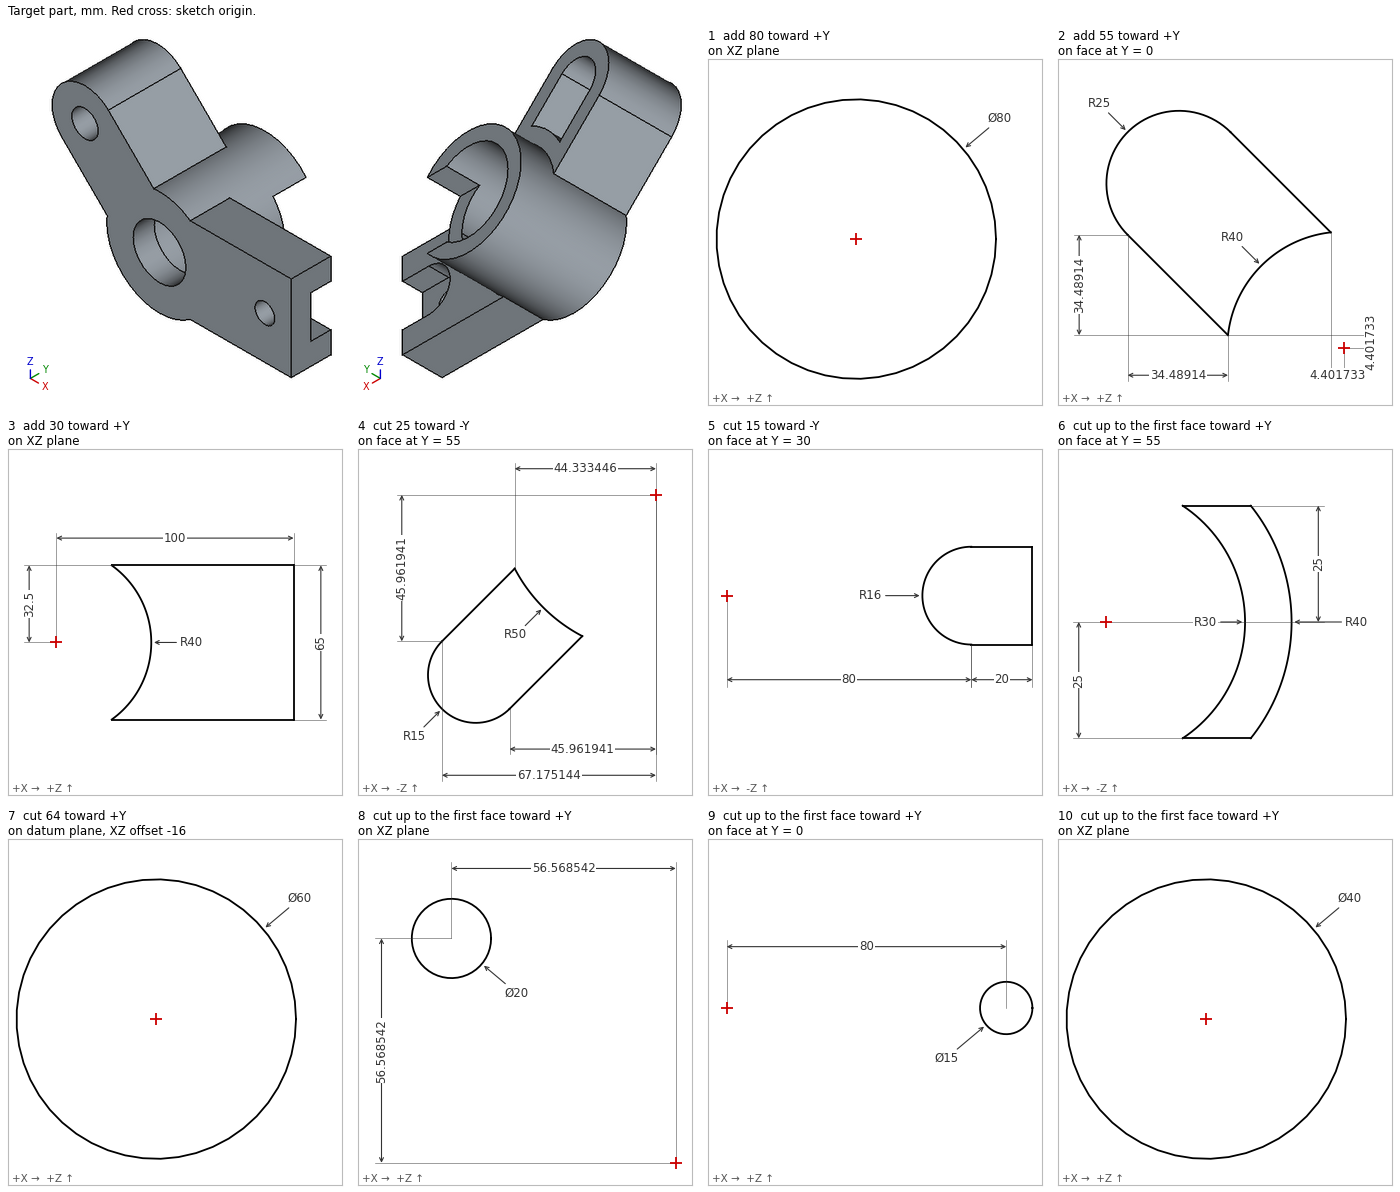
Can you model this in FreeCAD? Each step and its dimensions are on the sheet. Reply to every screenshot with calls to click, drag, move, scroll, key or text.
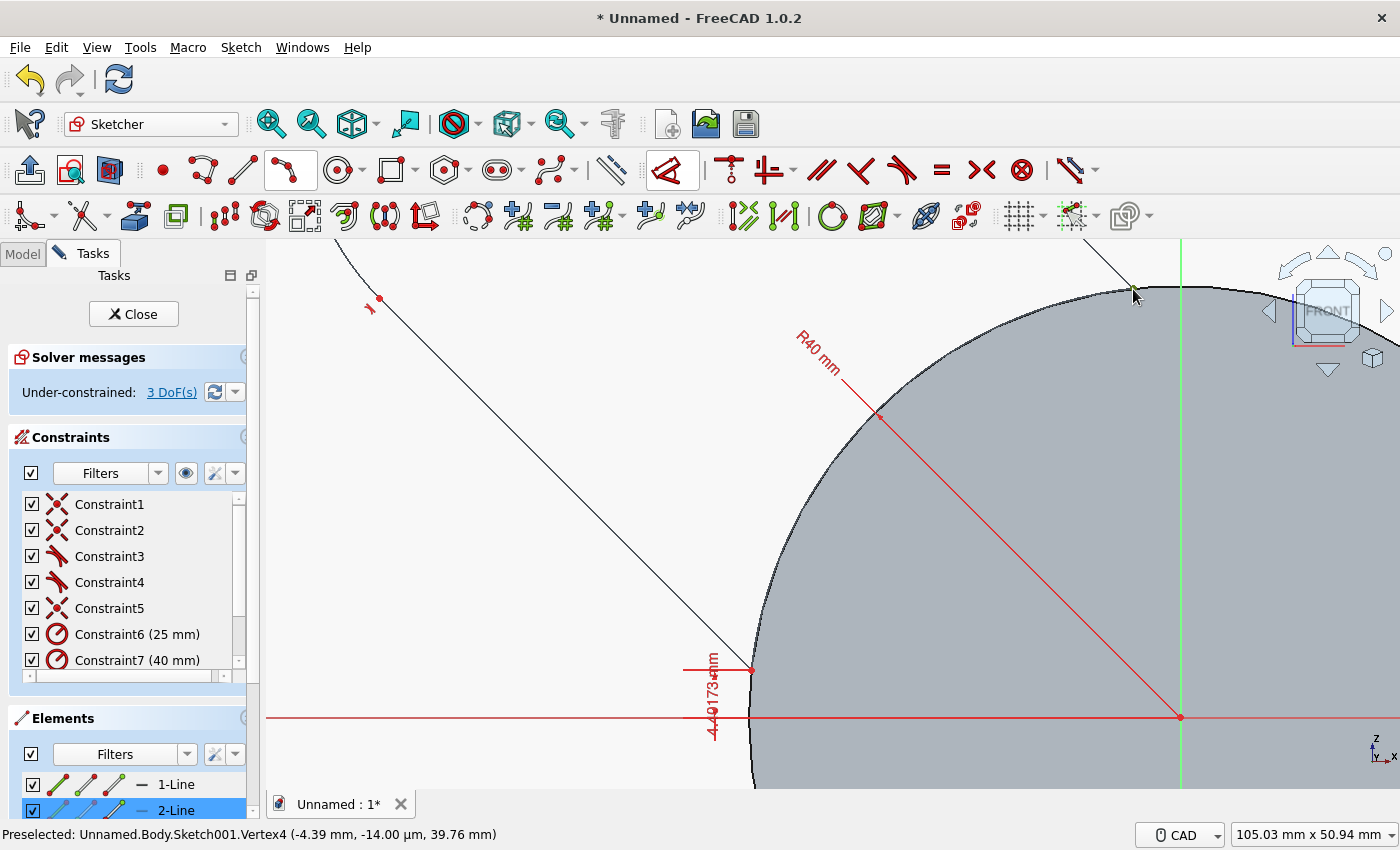
key(l)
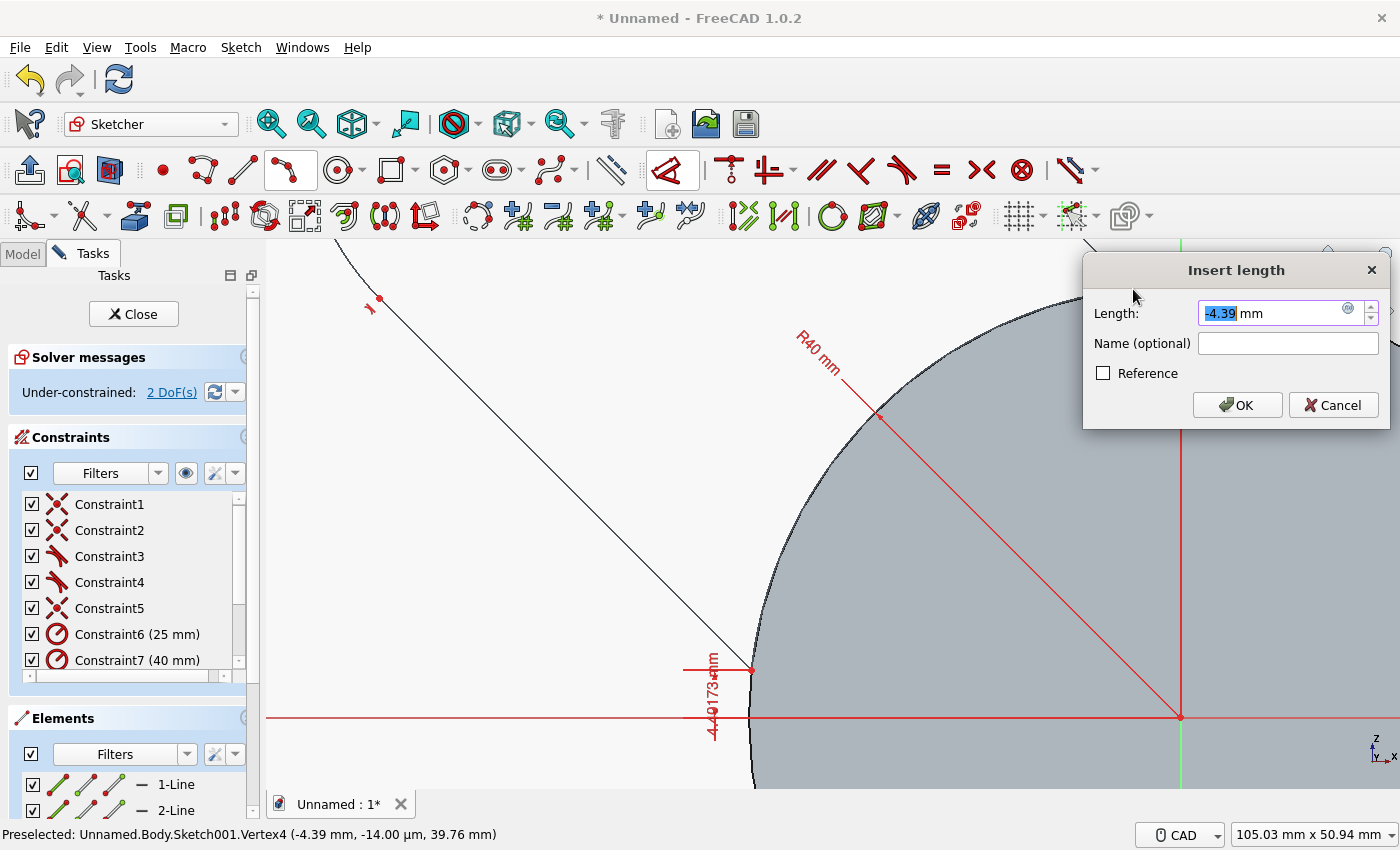
text(-4.401733)
key(Return)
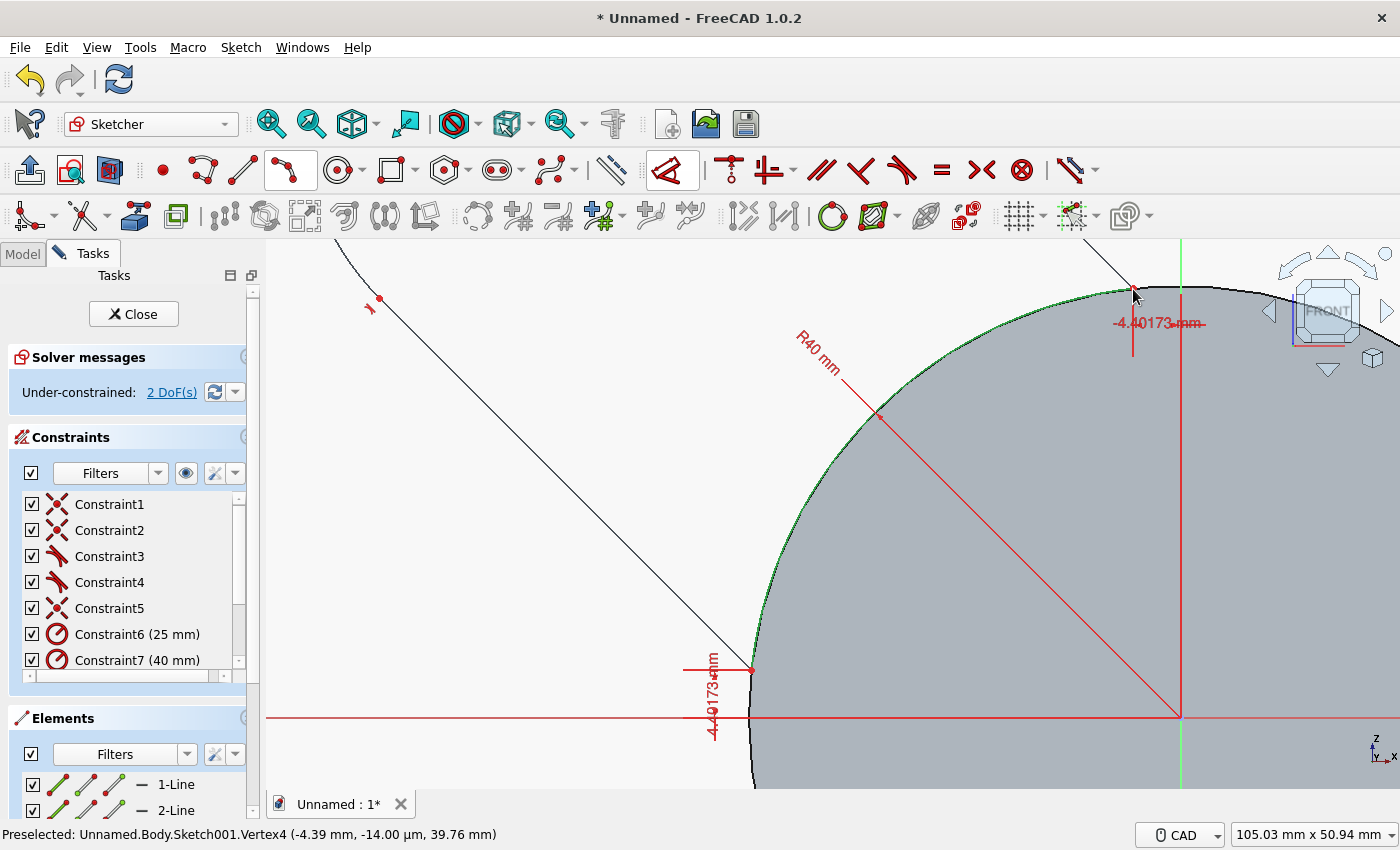
click(640, 559)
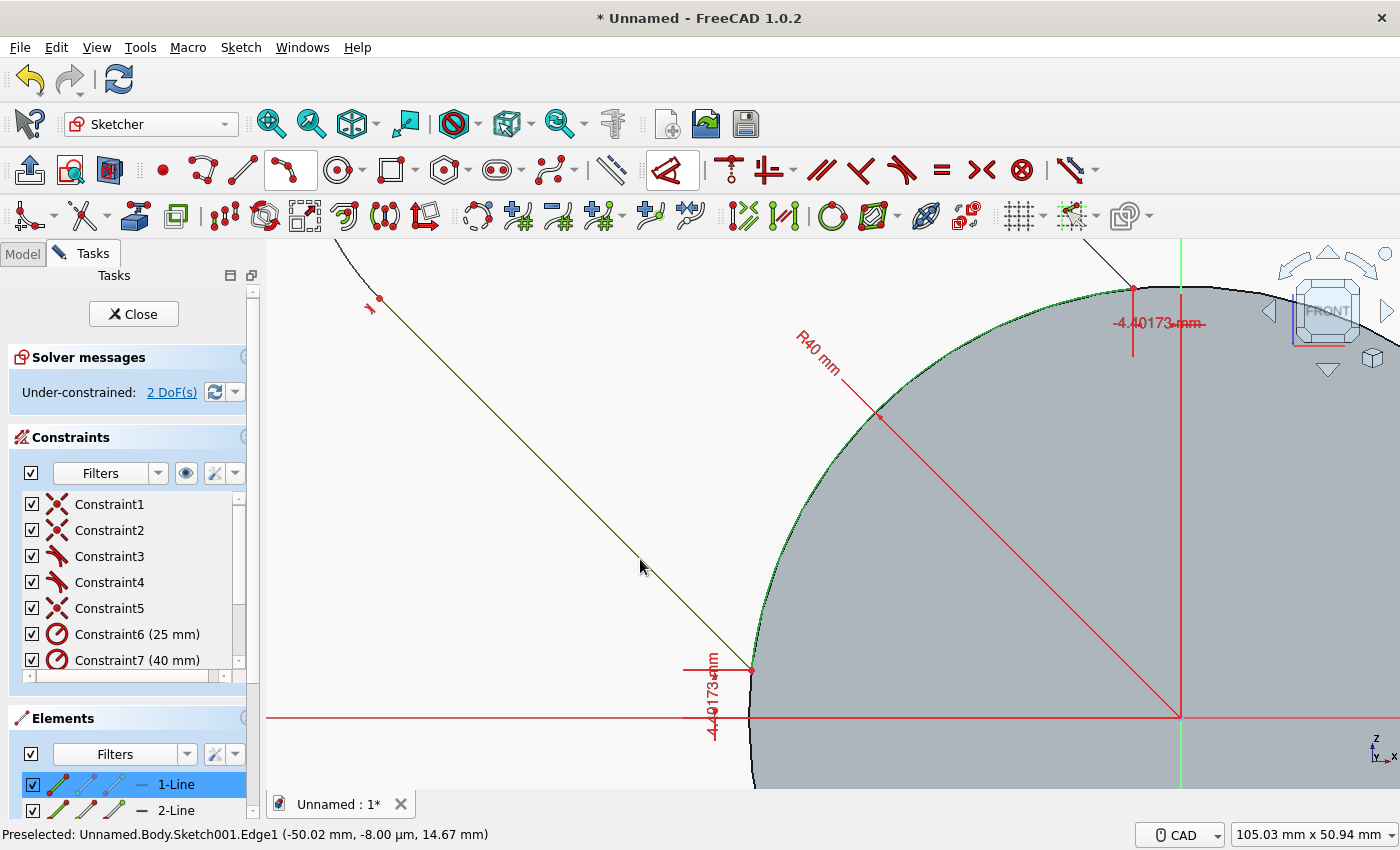
click(694, 170)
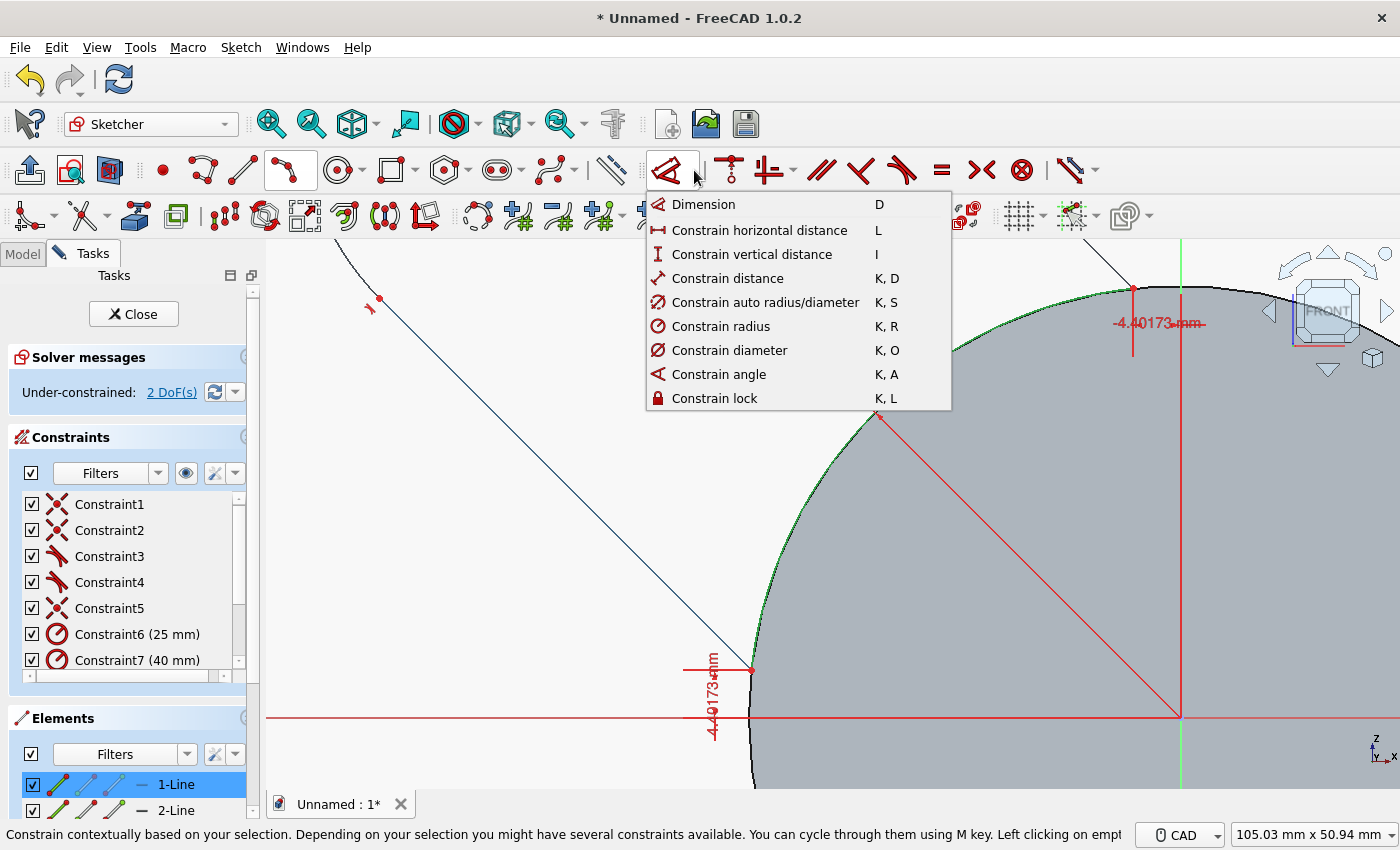
click(799, 230)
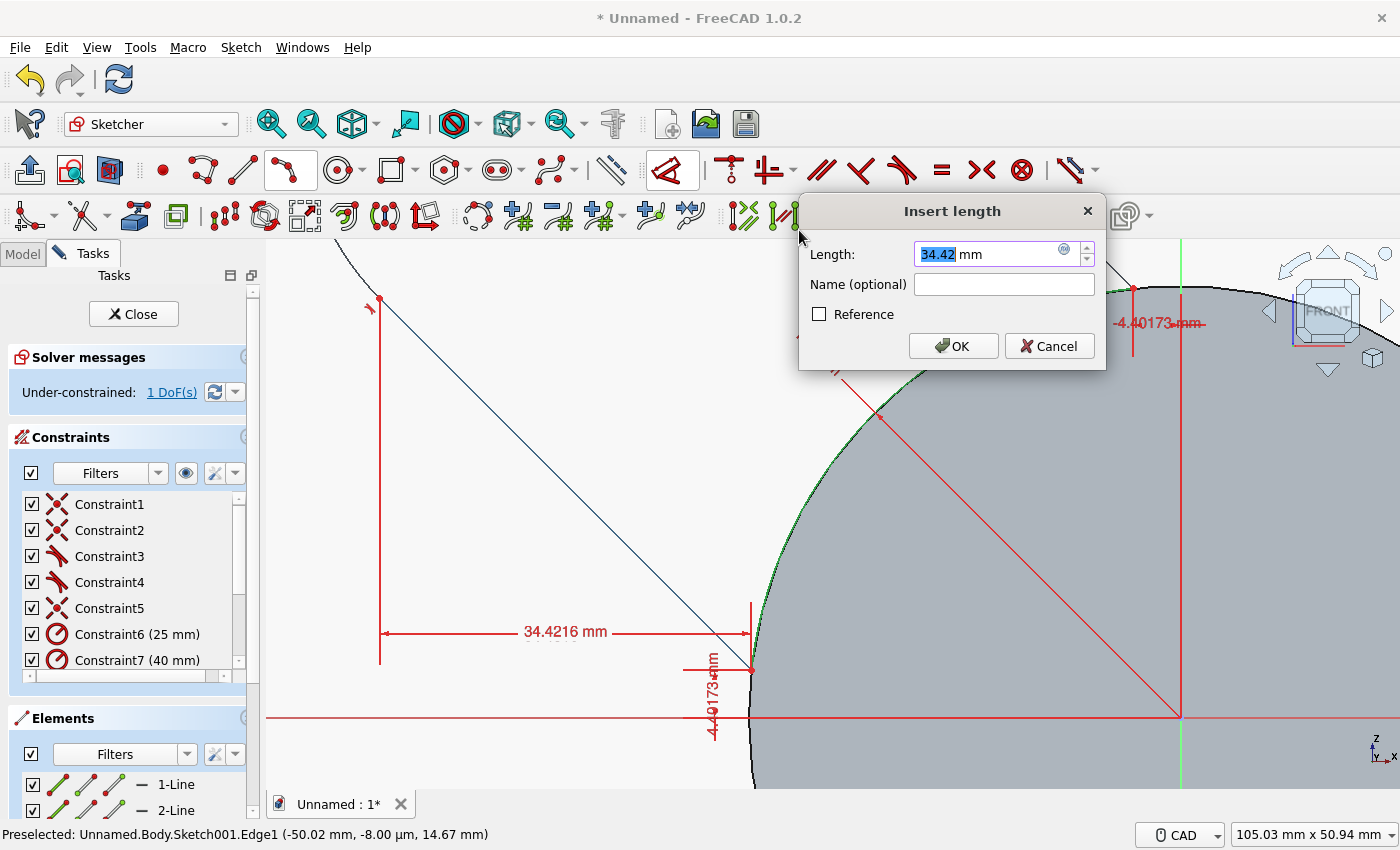
text(34.48914)
key(Return)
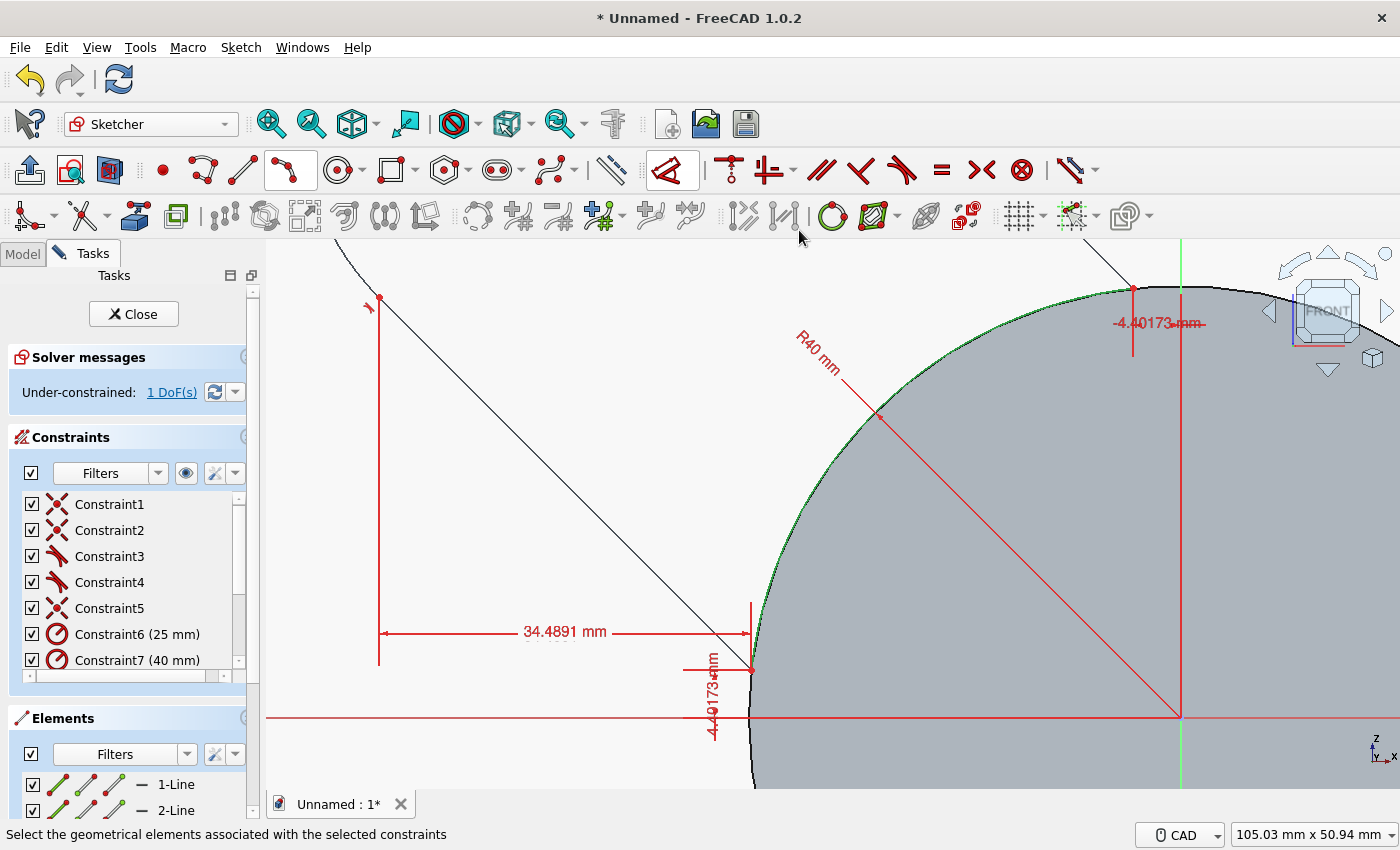
click(640, 559)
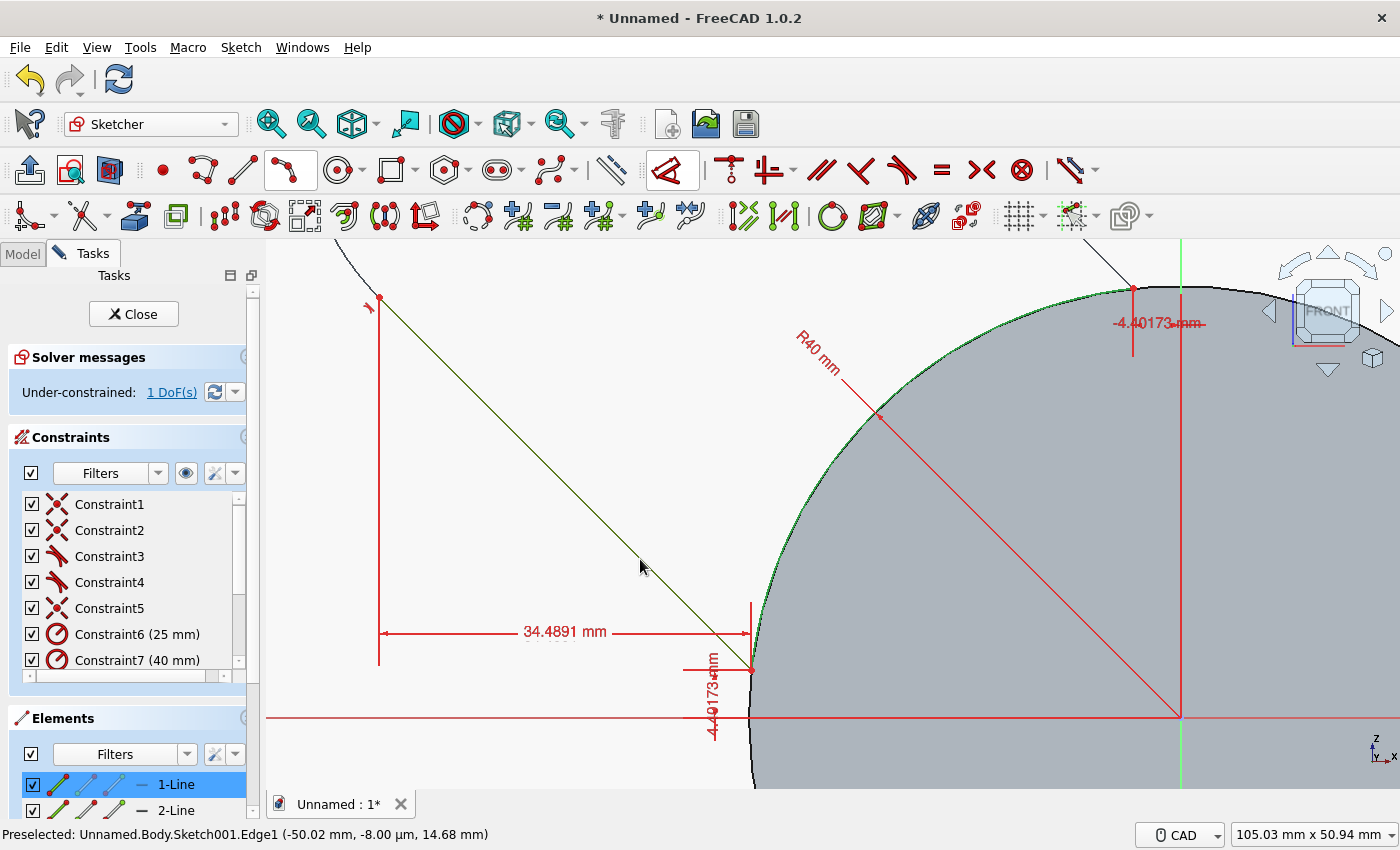
key(i)